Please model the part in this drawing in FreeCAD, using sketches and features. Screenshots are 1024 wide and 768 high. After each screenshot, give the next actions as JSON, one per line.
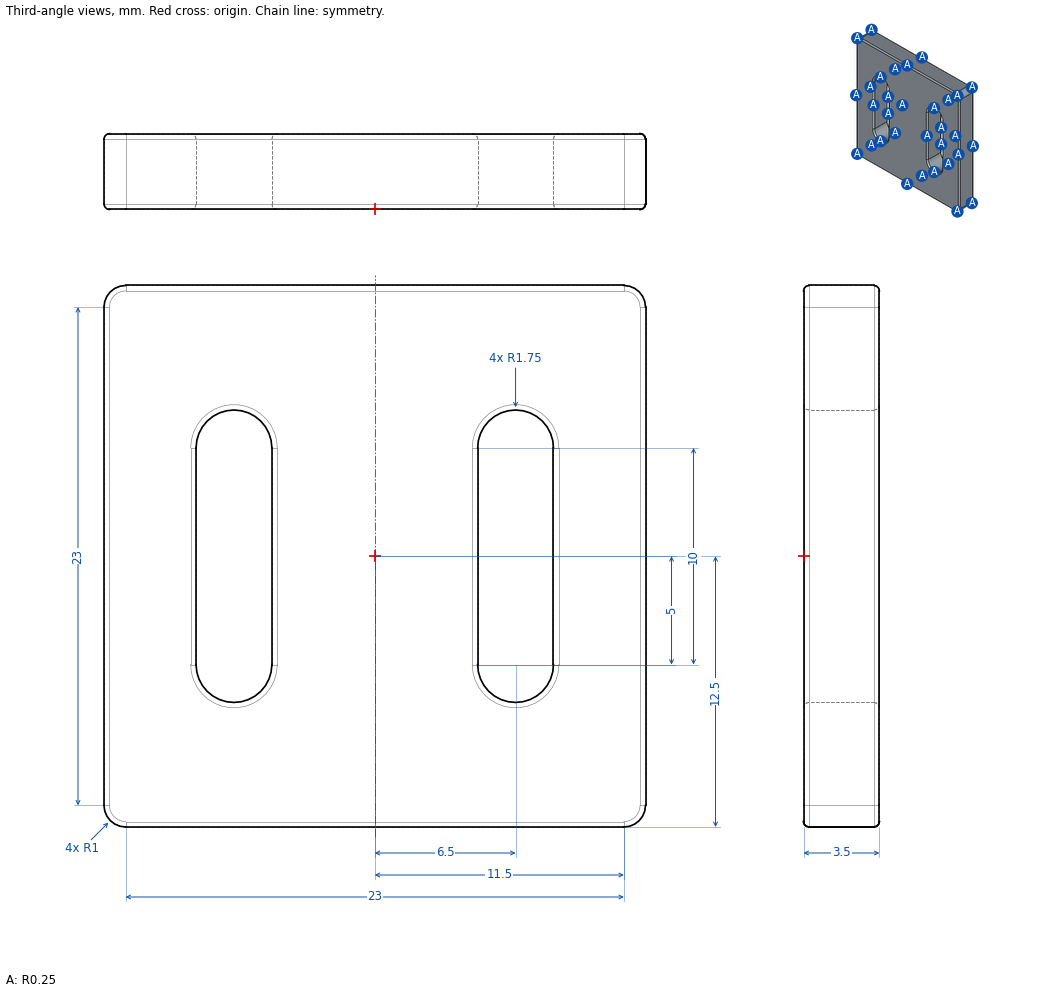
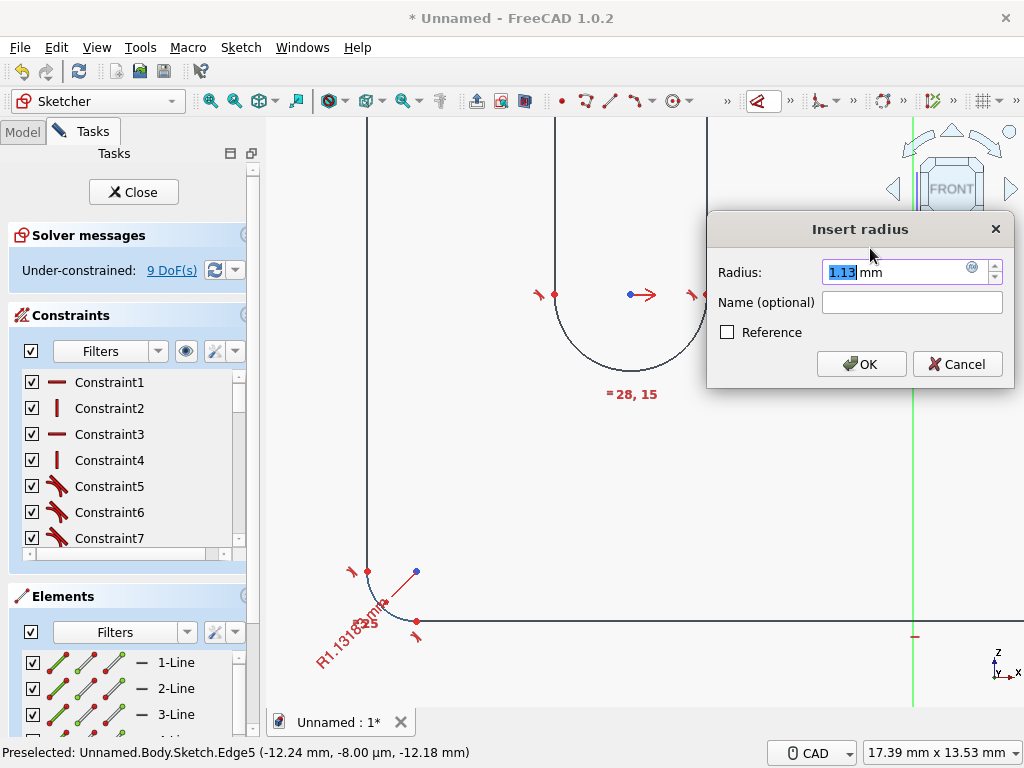
{"action": "type", "text": "1"}
{"action": "key", "text": "Return"}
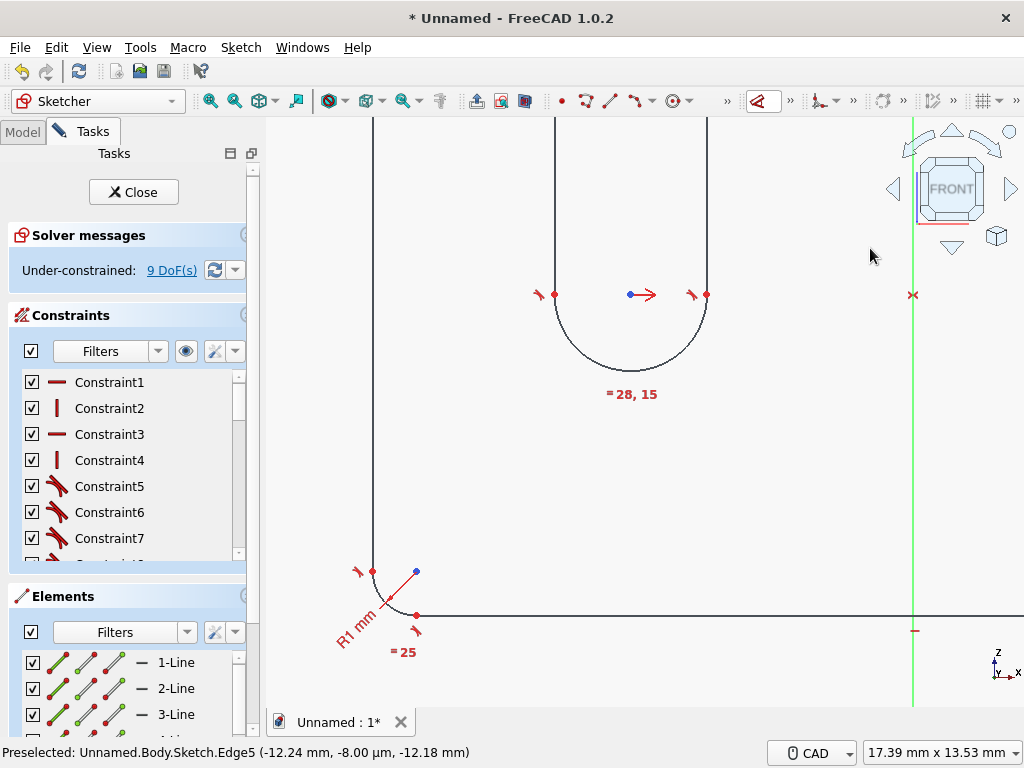
{"action": "scroll", "coordinate": [381, 609], "scroll_direction": "down", "scroll_amount": 5}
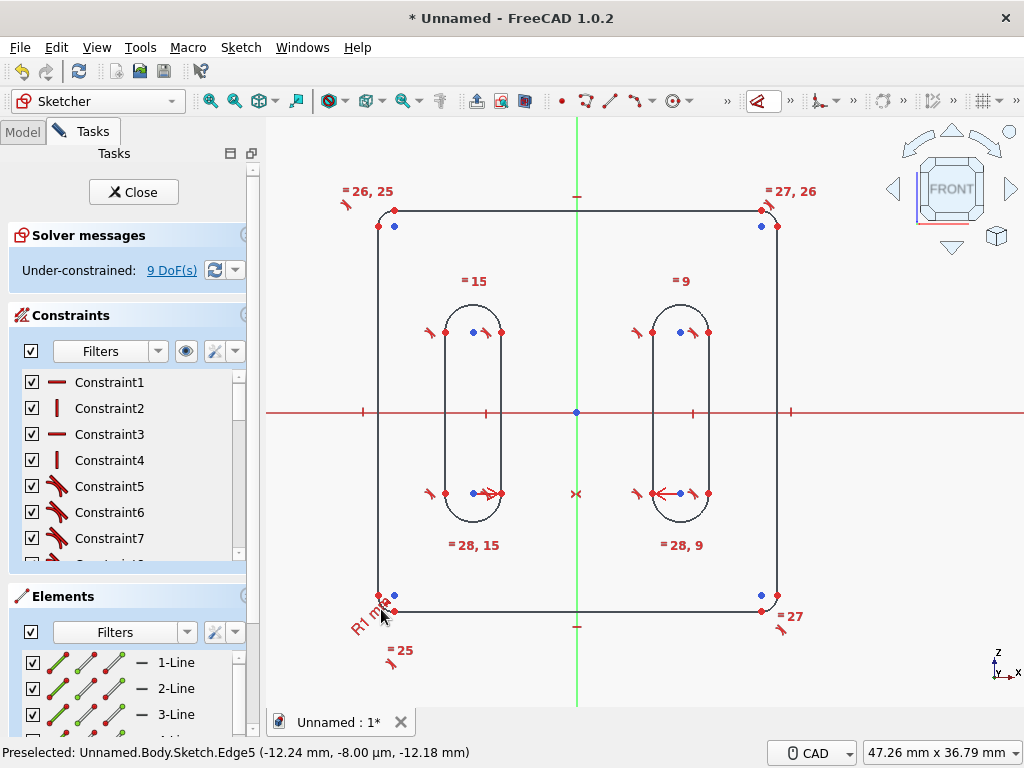
{"action": "scroll", "coordinate": [664, 517], "scroll_direction": "up", "scroll_amount": 2}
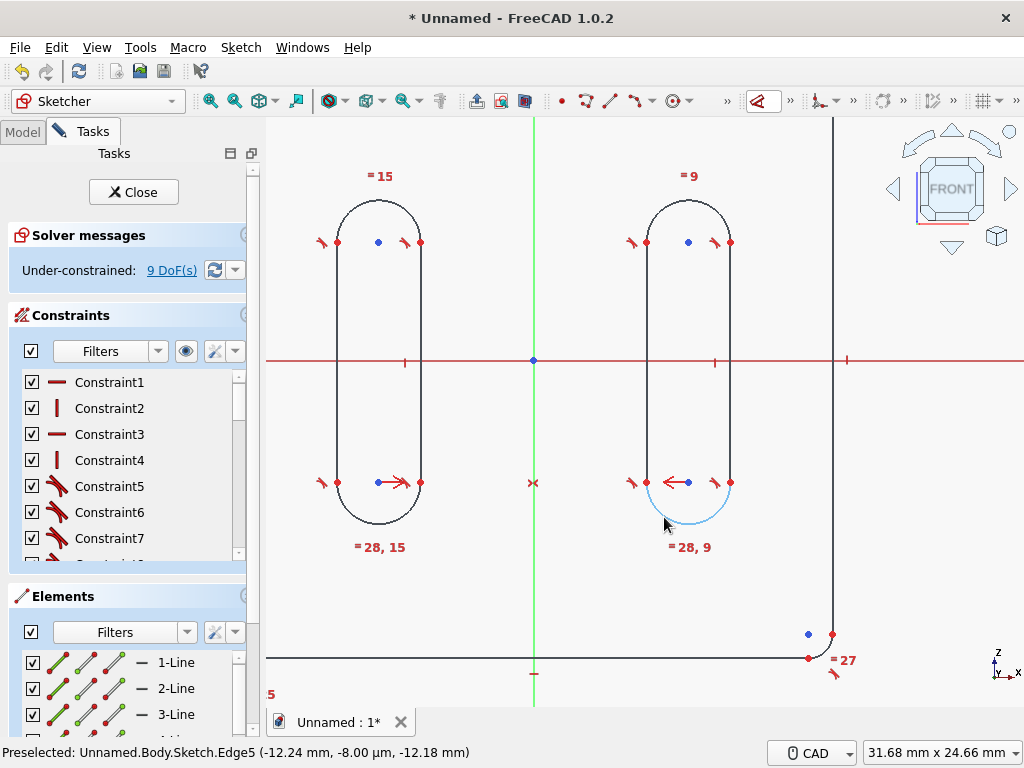
{"action": "left_click", "coordinate": [664, 516]}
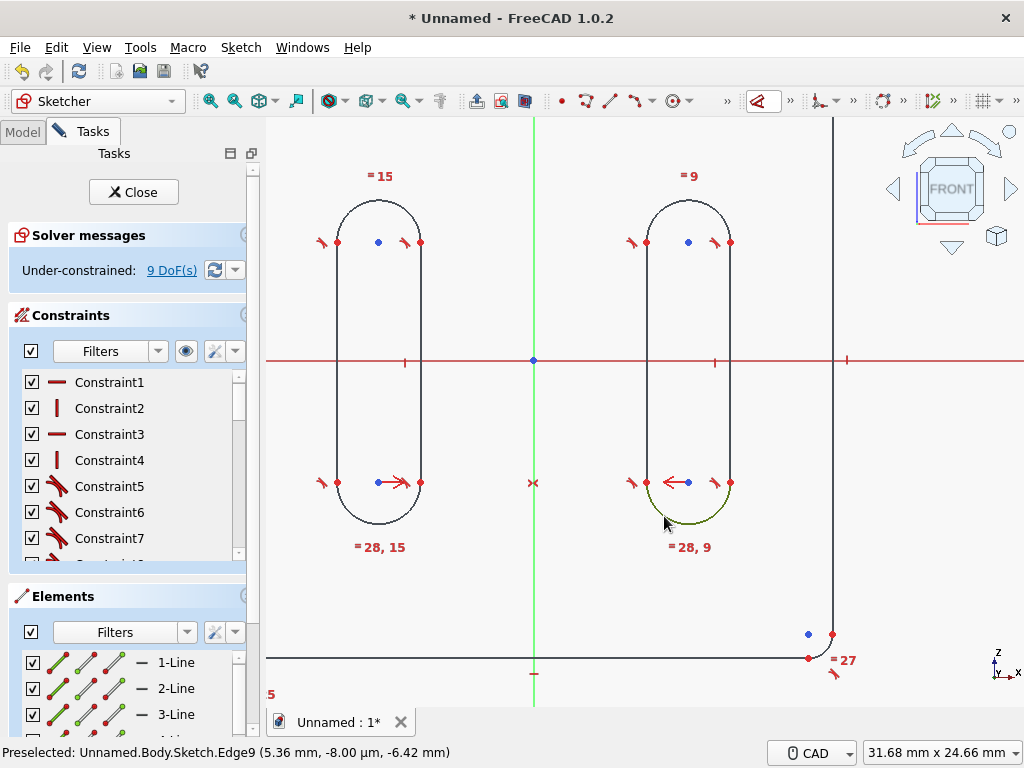
{"action": "key", "text": "k r"}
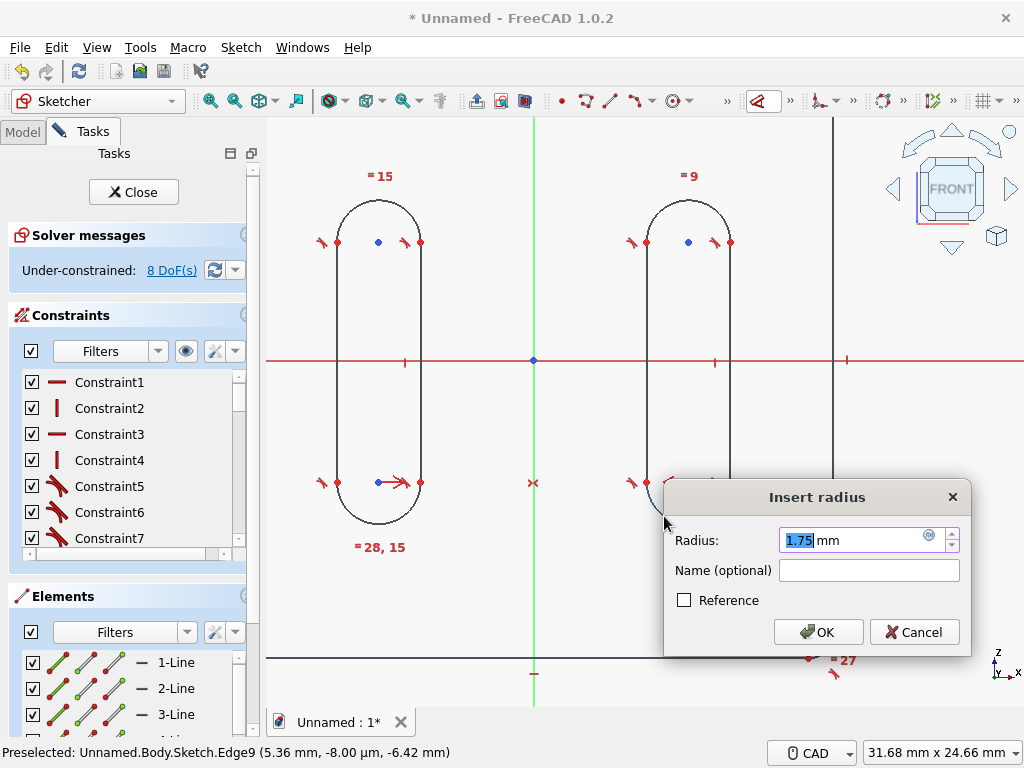
{"action": "type", "text": "1.75"}
{"action": "key", "text": "Return"}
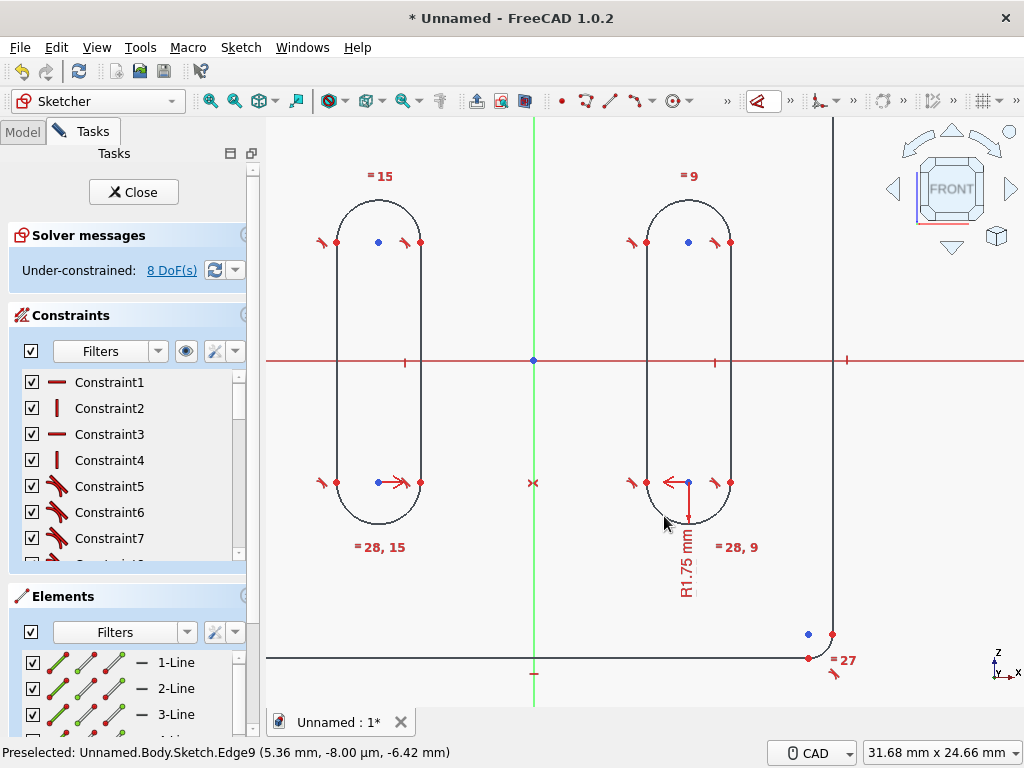
{"action": "left_click", "coordinate": [644, 658]}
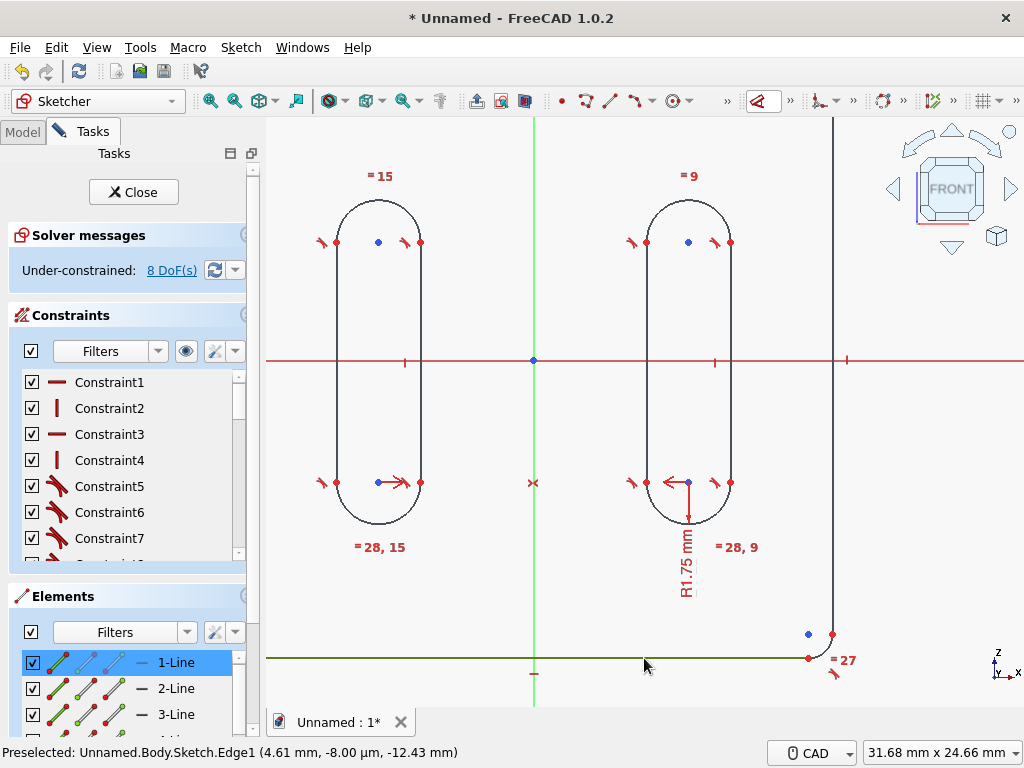
{"action": "key", "text": "l"}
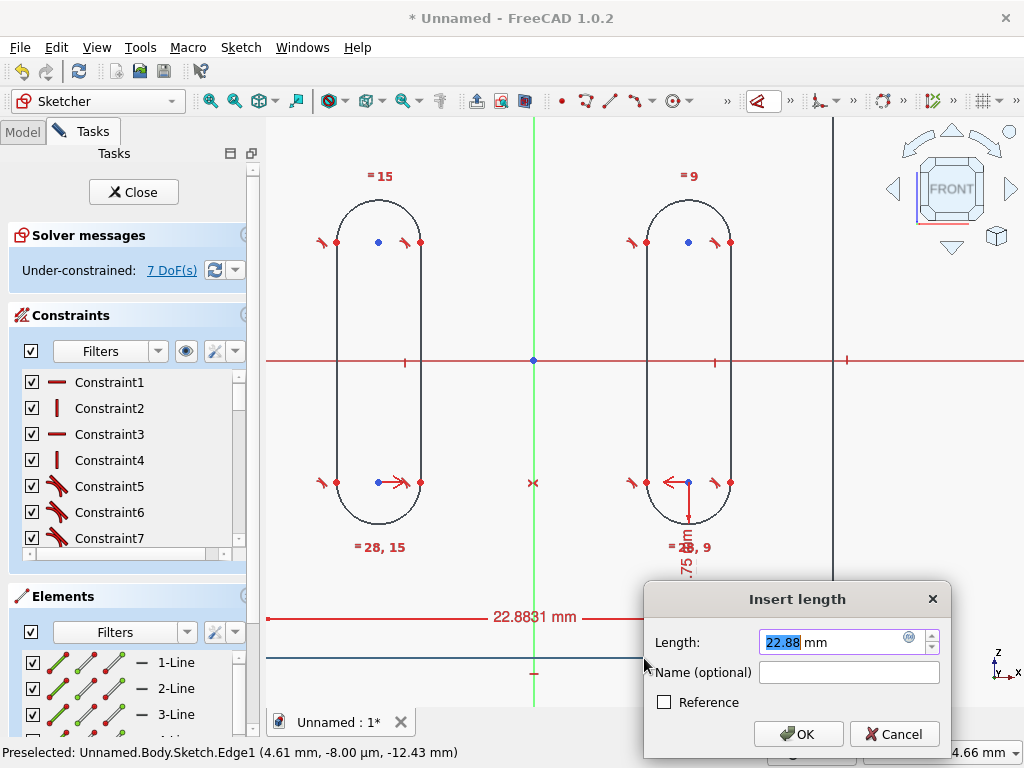
{"action": "type", "text": "23"}
{"action": "key", "text": "Return"}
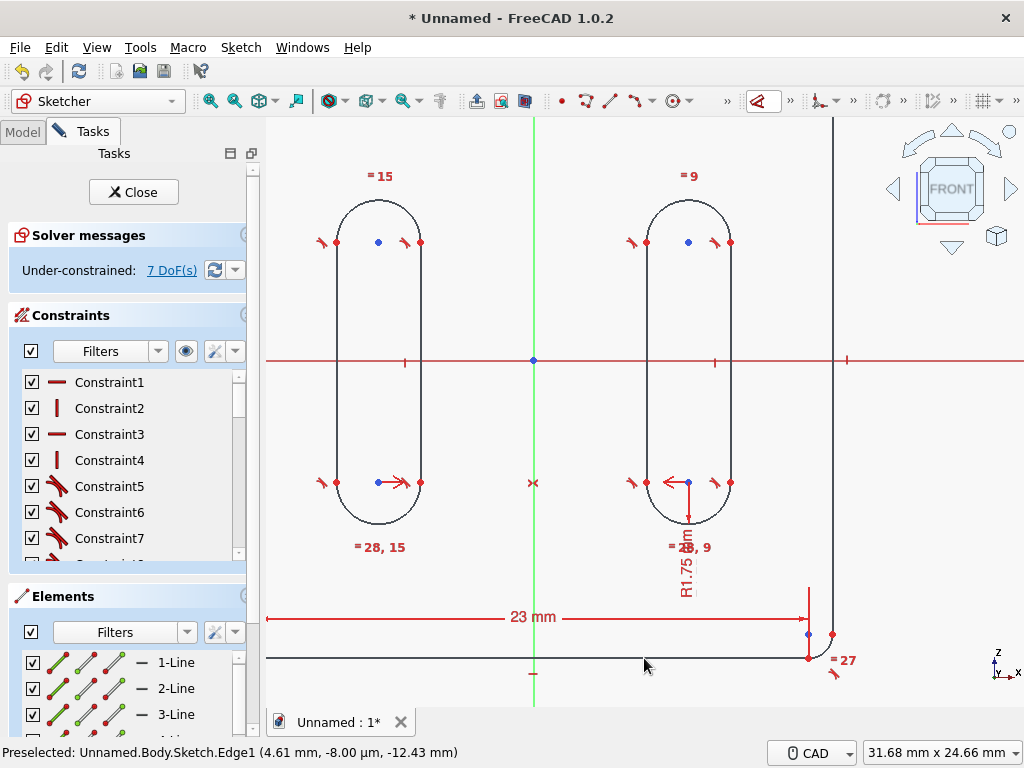
{"action": "scroll", "coordinate": [664, 516], "scroll_direction": "down", "scroll_amount": 2}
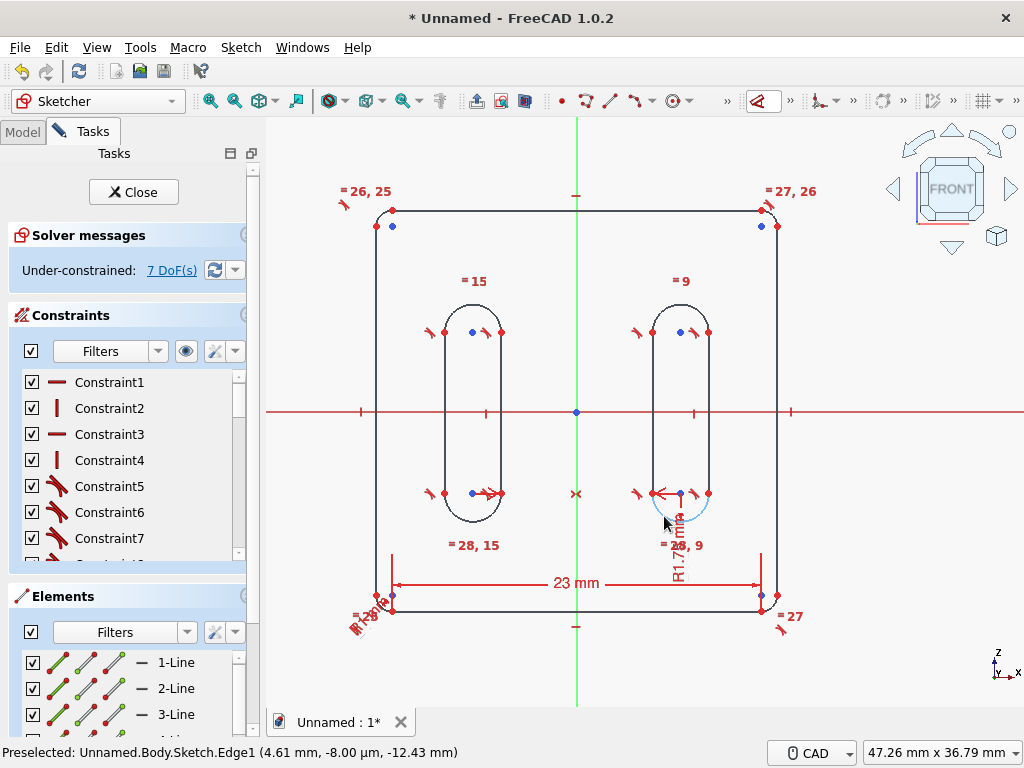
{"action": "left_click", "coordinate": [376, 485]}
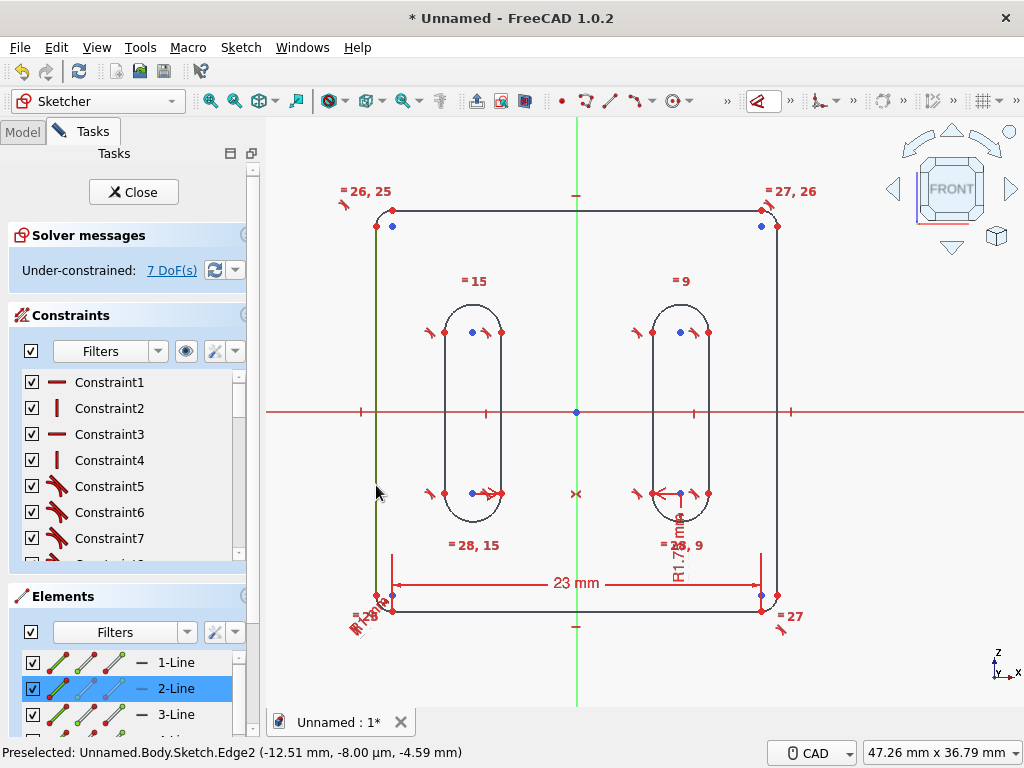
{"action": "key", "text": "i"}